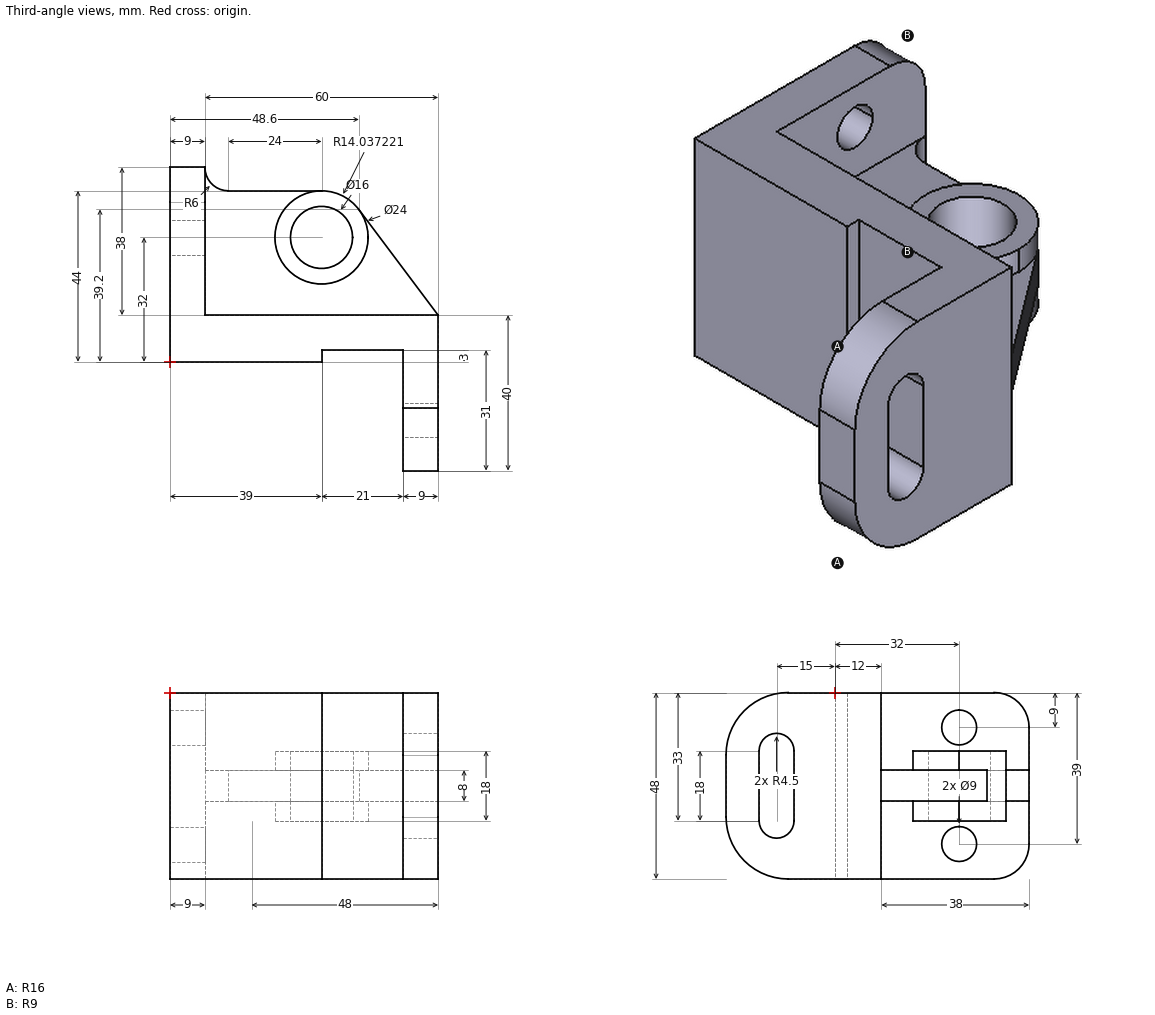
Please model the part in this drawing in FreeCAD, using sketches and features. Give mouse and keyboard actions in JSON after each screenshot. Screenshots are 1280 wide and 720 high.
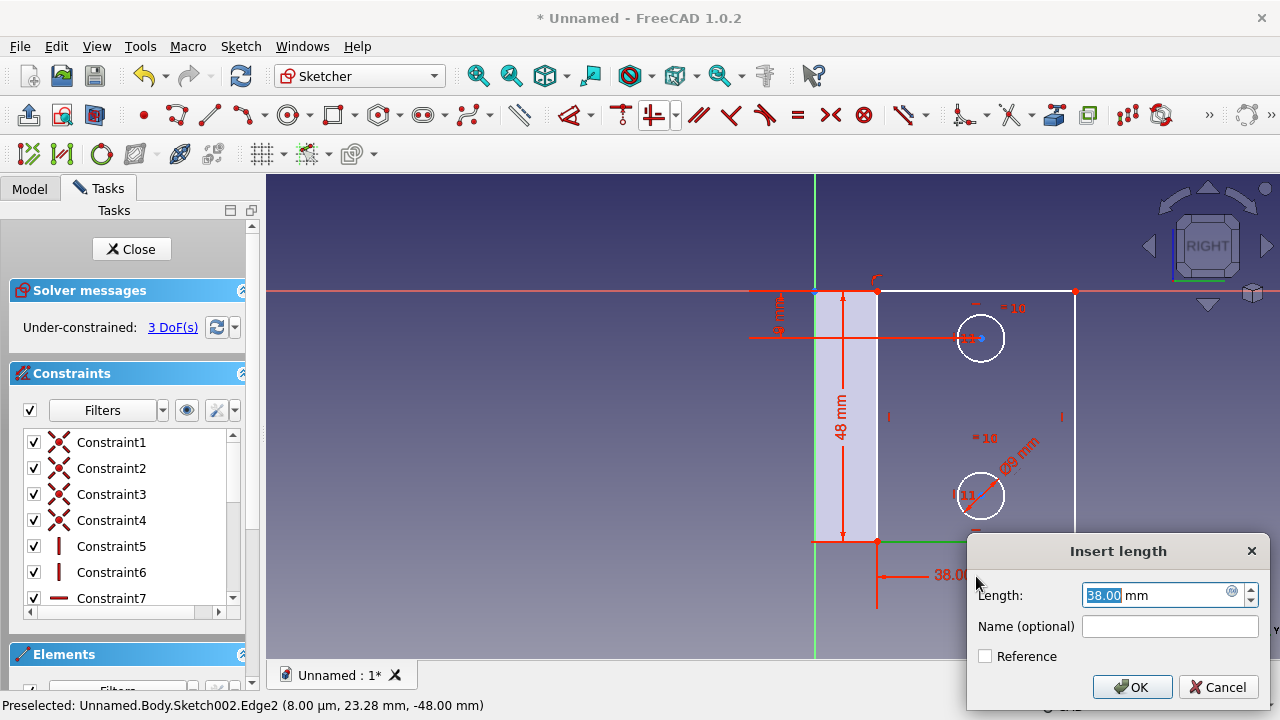
{"action": "type", "text": "38"}
{"action": "key", "text": "Return"}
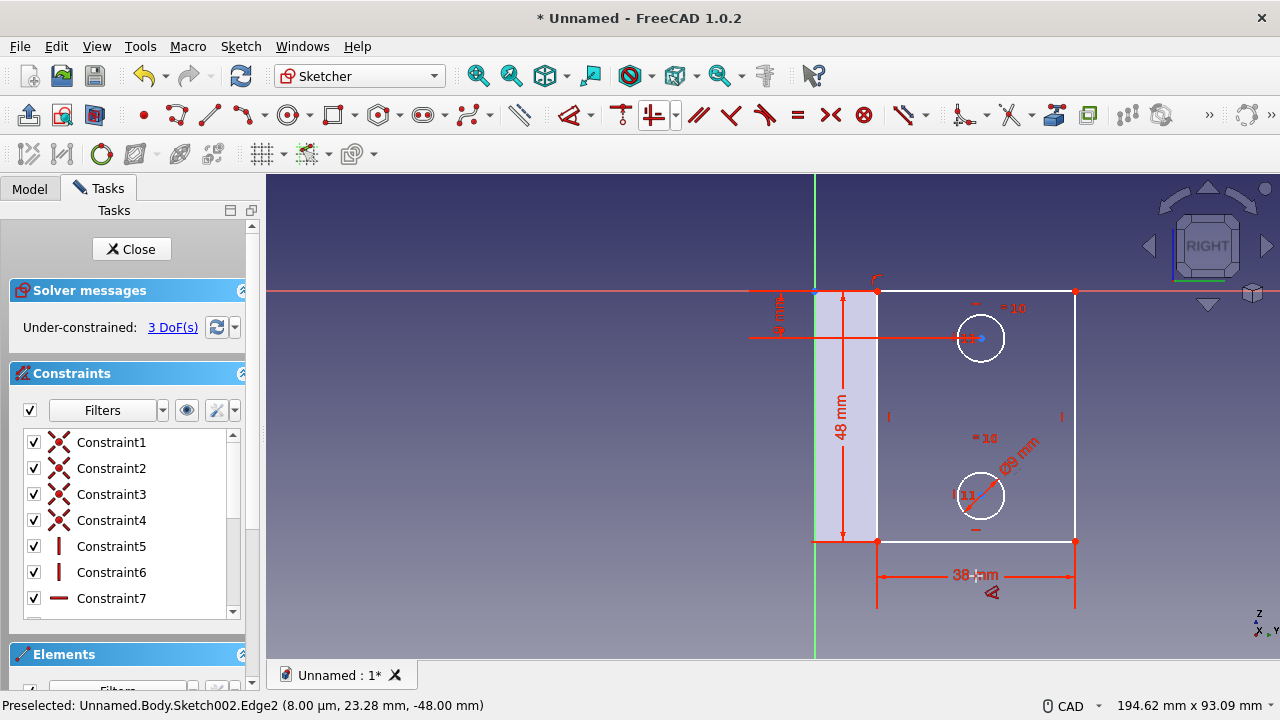
{"action": "left_click", "coordinate": [981, 496]}
{"action": "left_click", "coordinate": [898, 257]}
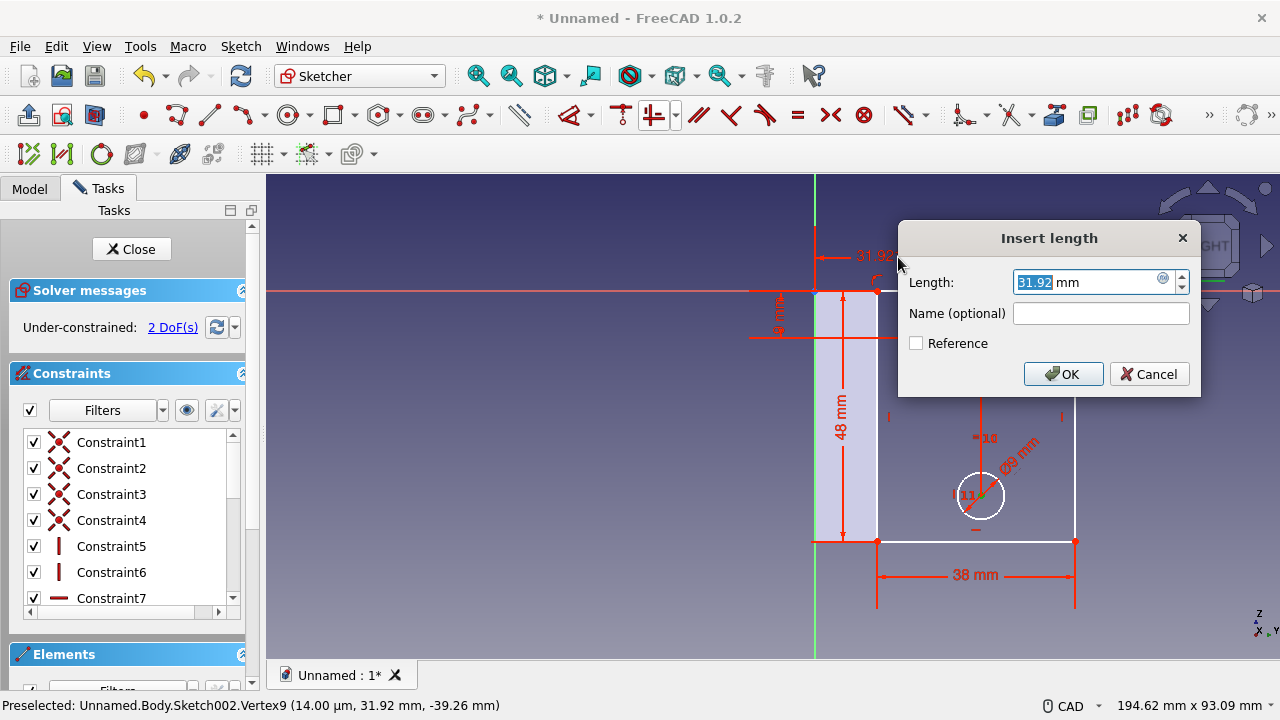
{"action": "type", "text": "32"}
{"action": "key", "text": "Return"}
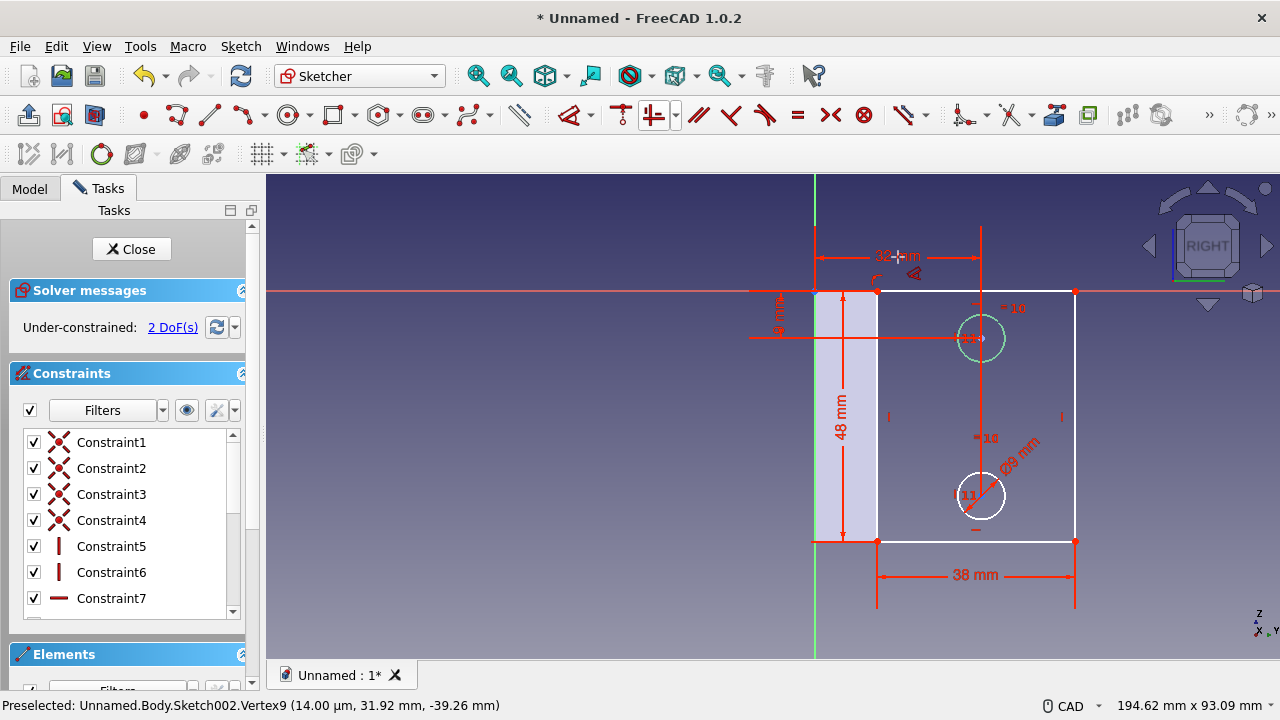
{"action": "left_click", "coordinate": [981, 496]}
{"action": "left_click", "coordinate": [781, 394]}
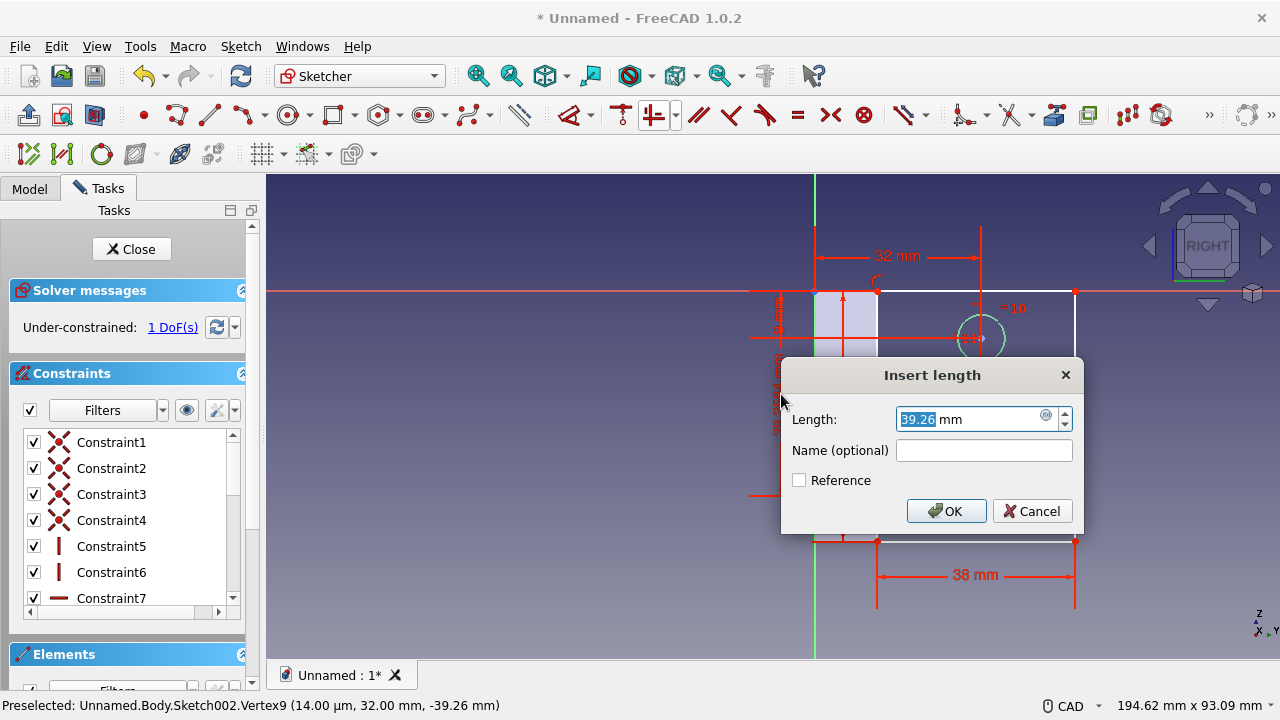
{"action": "type", "text": "39"}
{"action": "key", "text": "Return"}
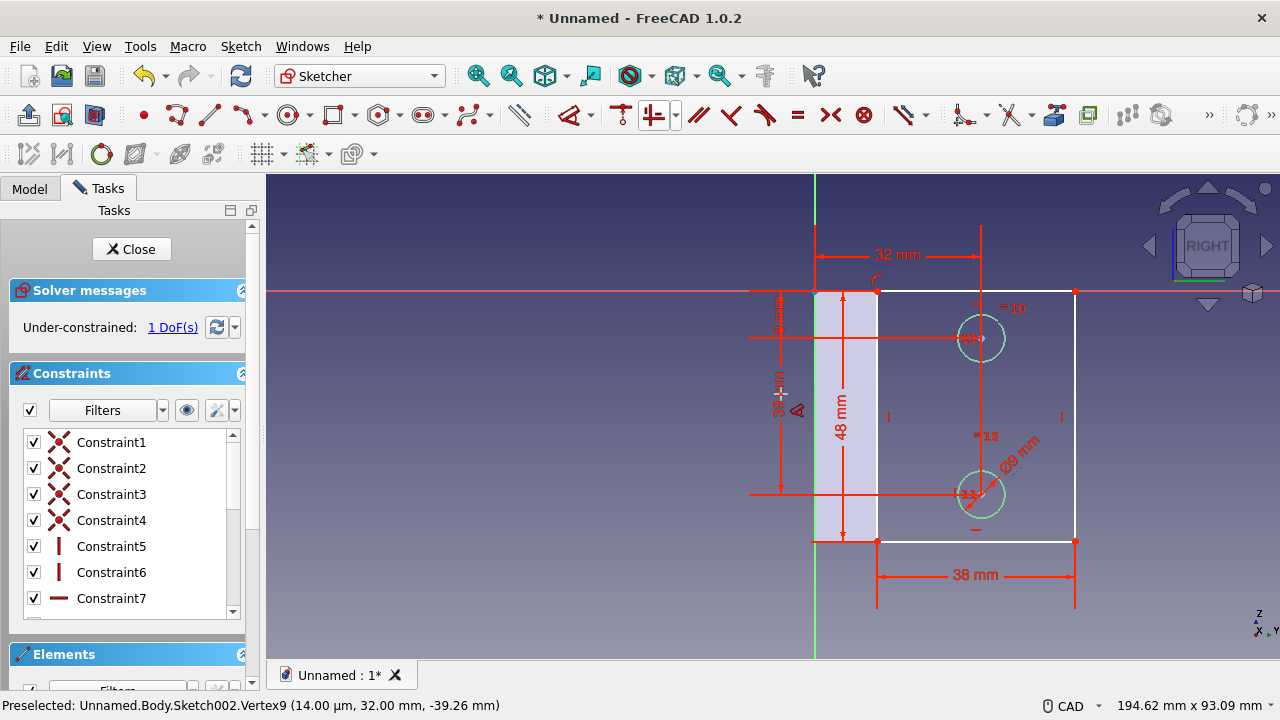
{"action": "left_click", "coordinate": [877, 291]}
{"action": "left_click", "coordinate": [860, 325]}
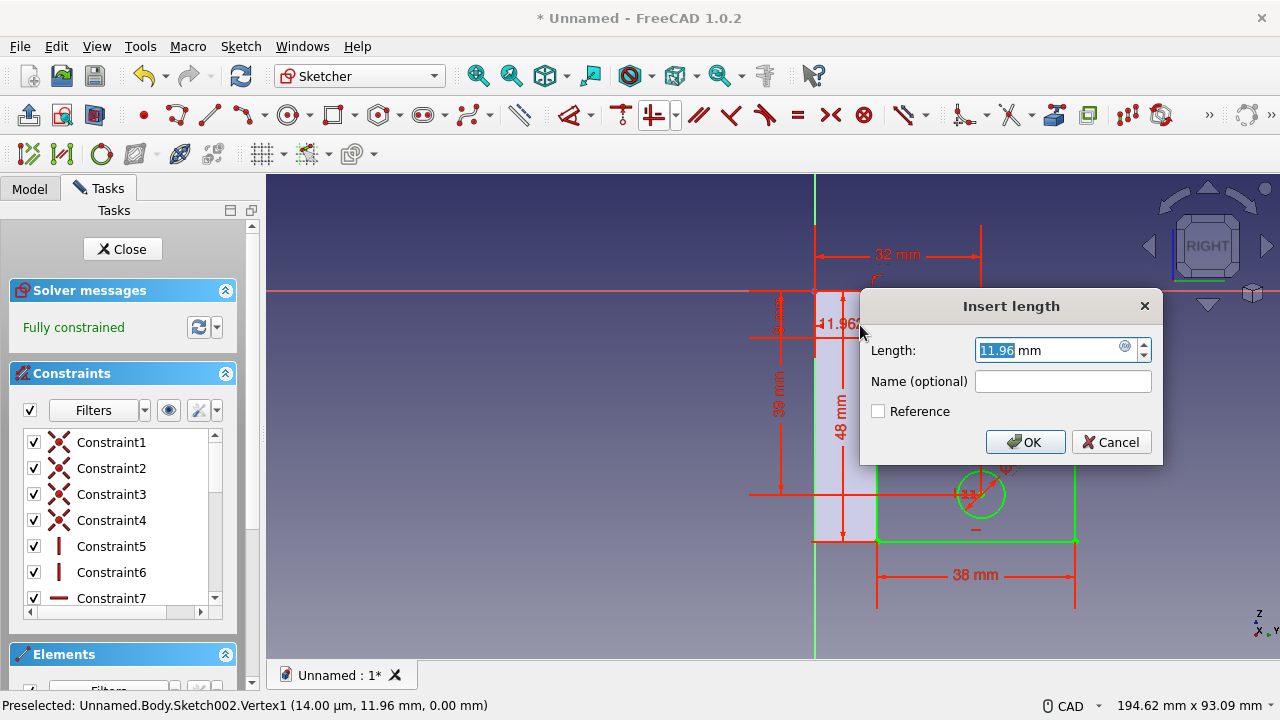
{"action": "type", "text": "12"}
{"action": "key", "text": "Return"}
{"action": "key", "text": "Escape"}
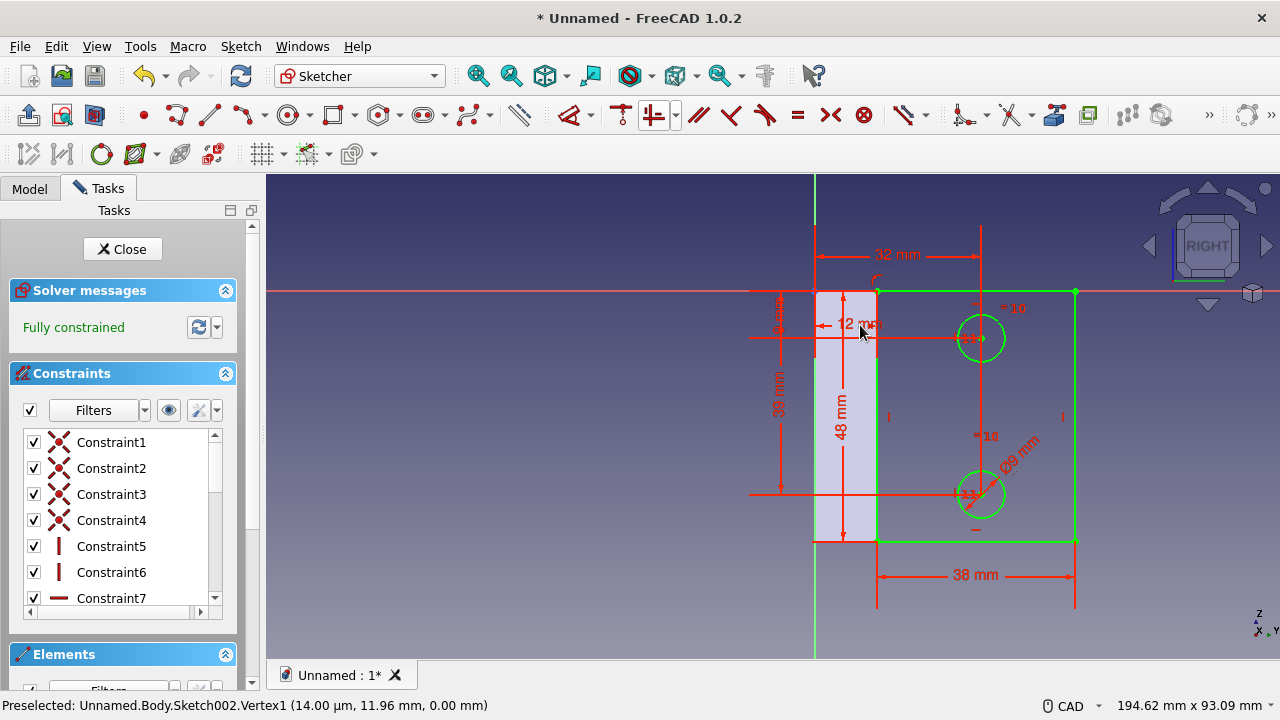
{"action": "left_click", "coordinate": [123, 249]}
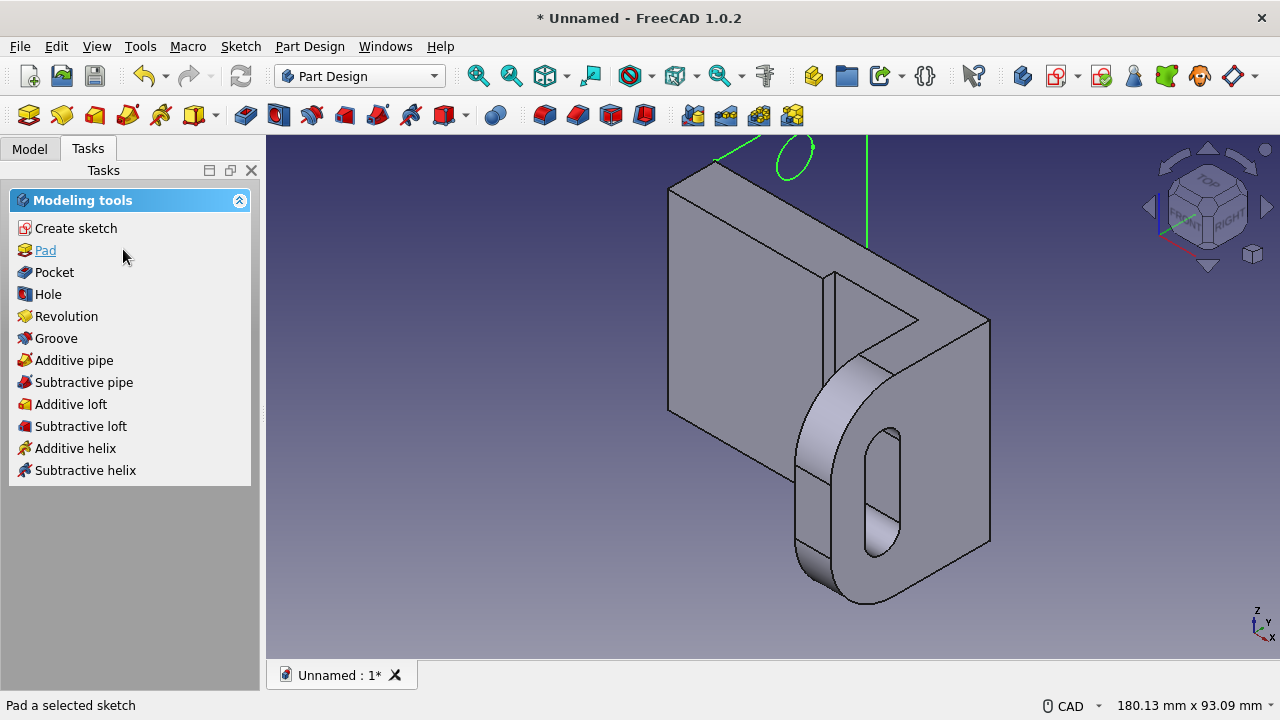
{"action": "left_click", "coordinate": [29, 116]}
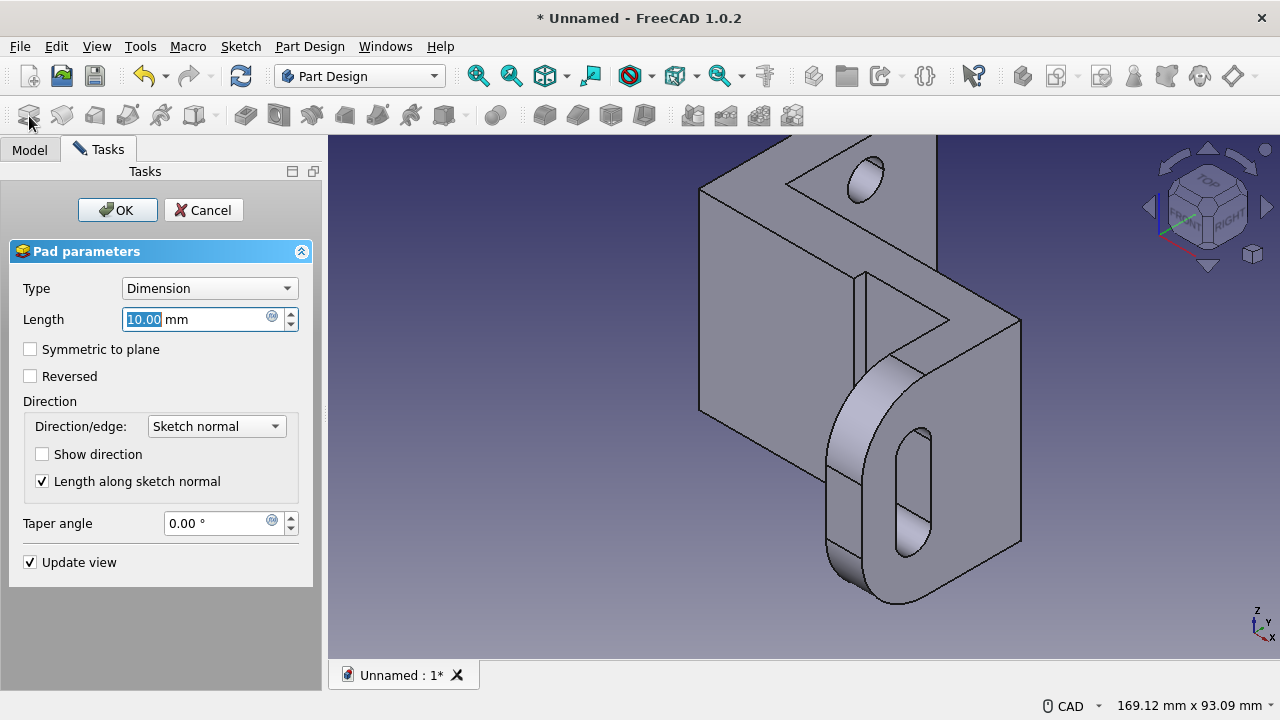
{"action": "type", "text": "9"}
{"action": "key", "text": "Tab"}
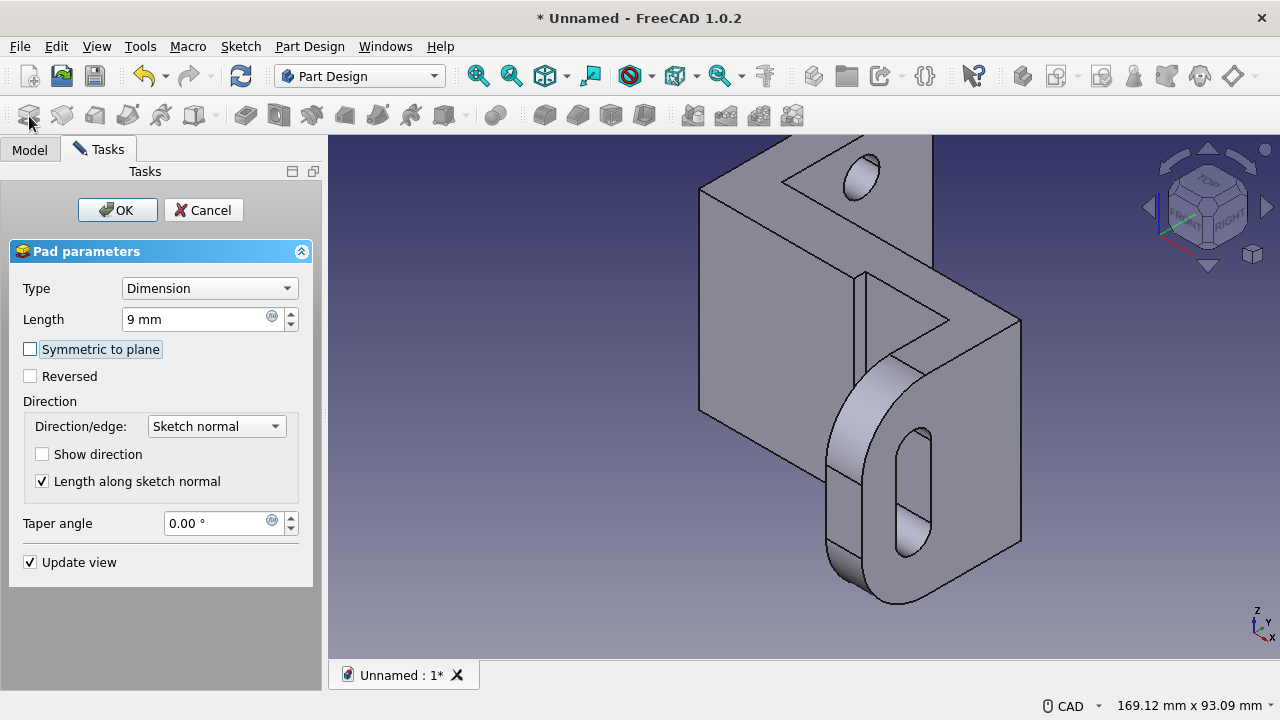
{"action": "left_click", "coordinate": [118, 210]}